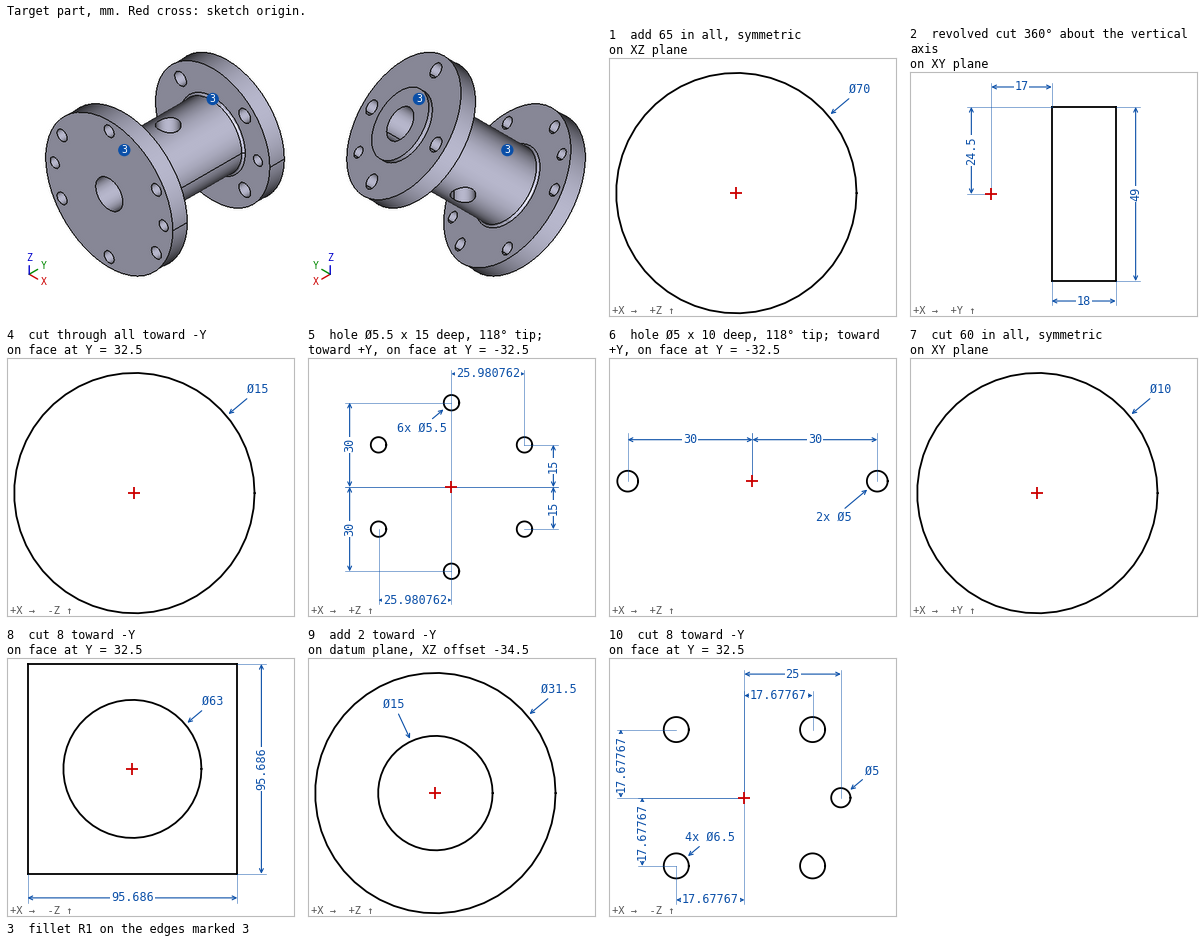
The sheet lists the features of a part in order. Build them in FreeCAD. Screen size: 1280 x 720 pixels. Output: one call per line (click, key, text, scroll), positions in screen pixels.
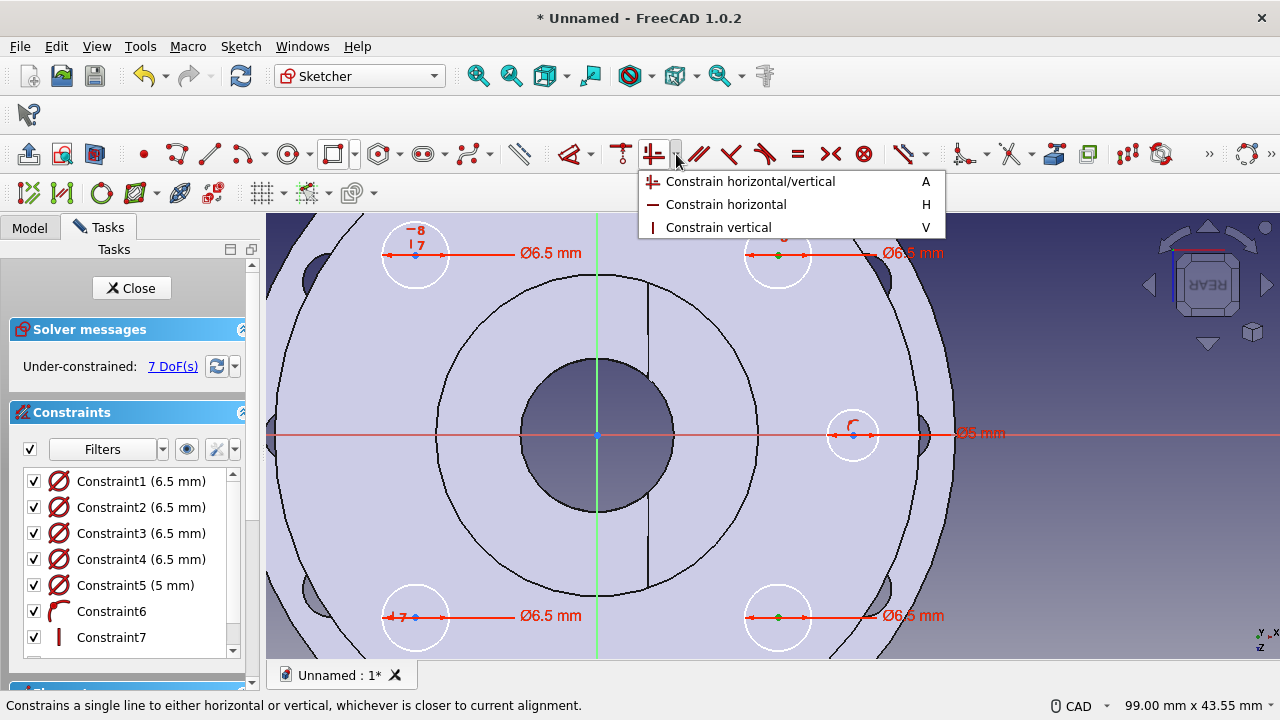
click(792, 228)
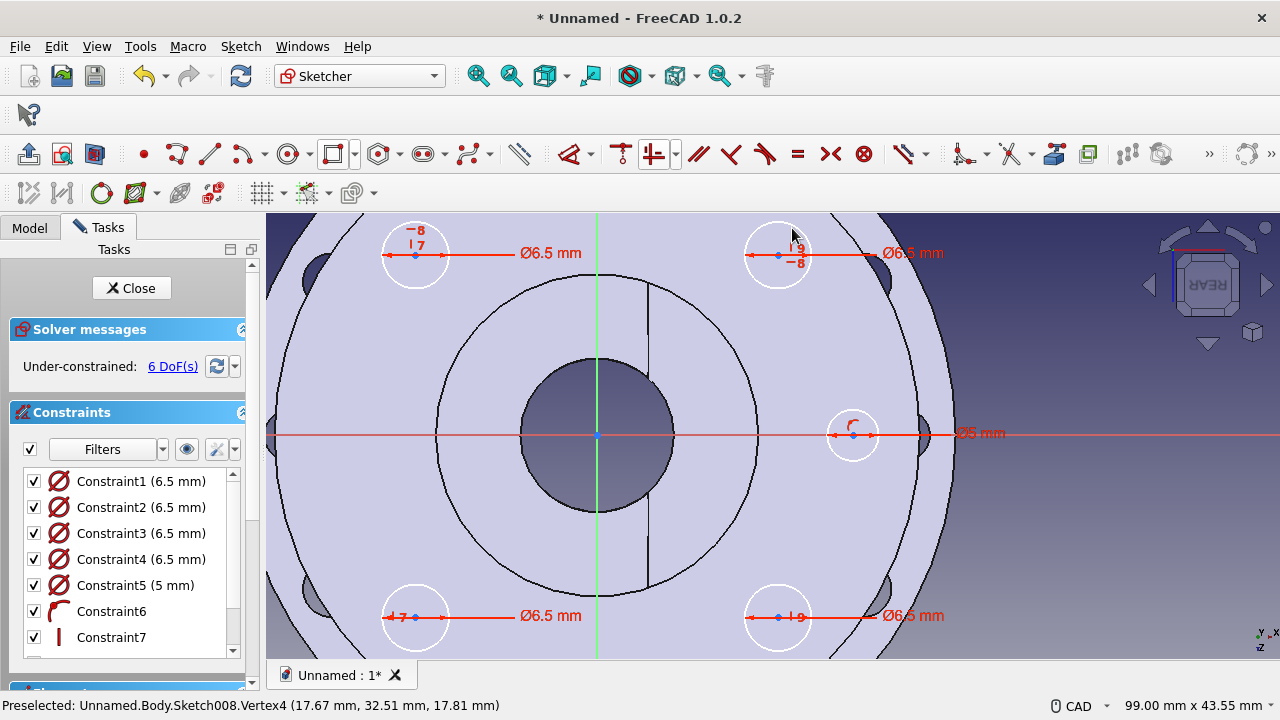
click(416, 618)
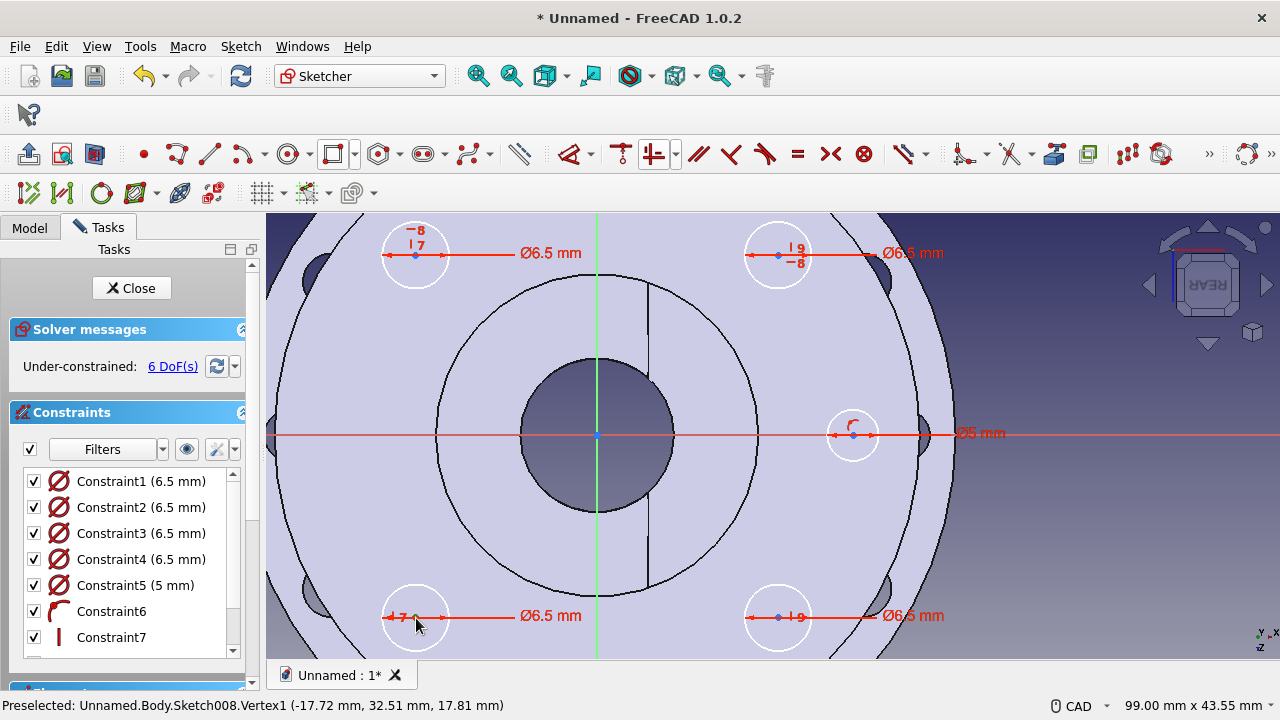
click(778, 618)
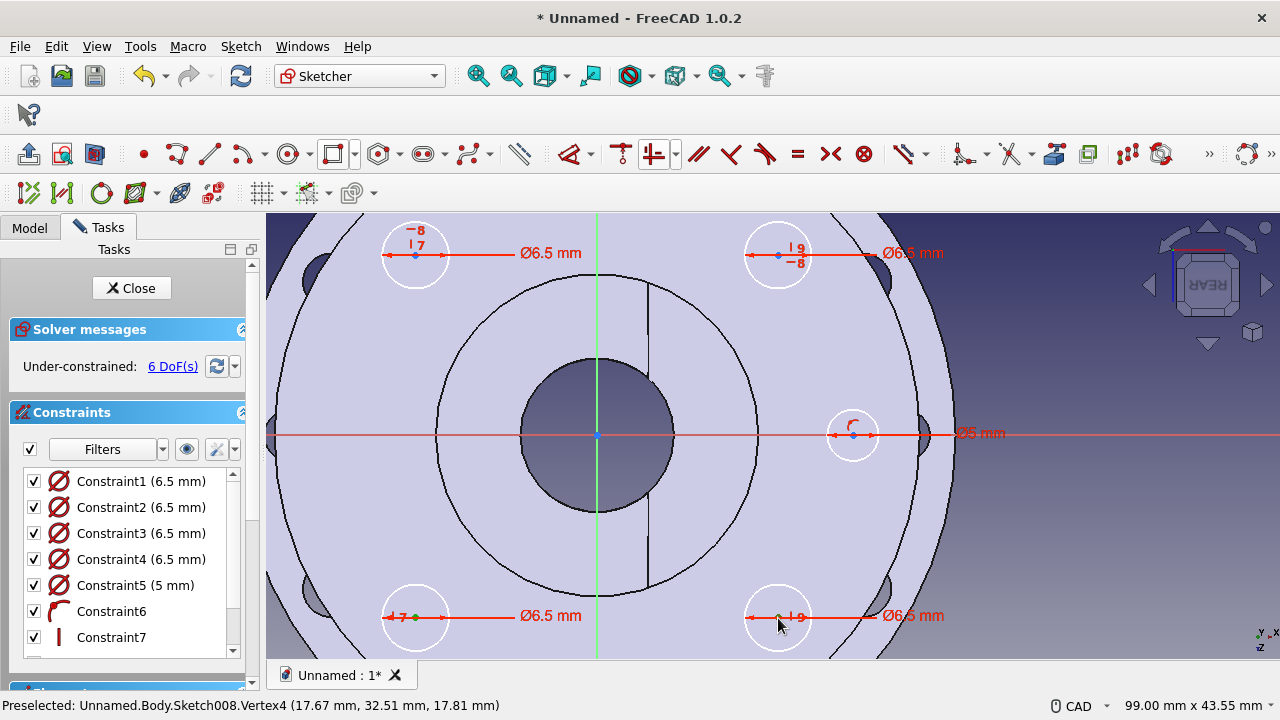
click(676, 154)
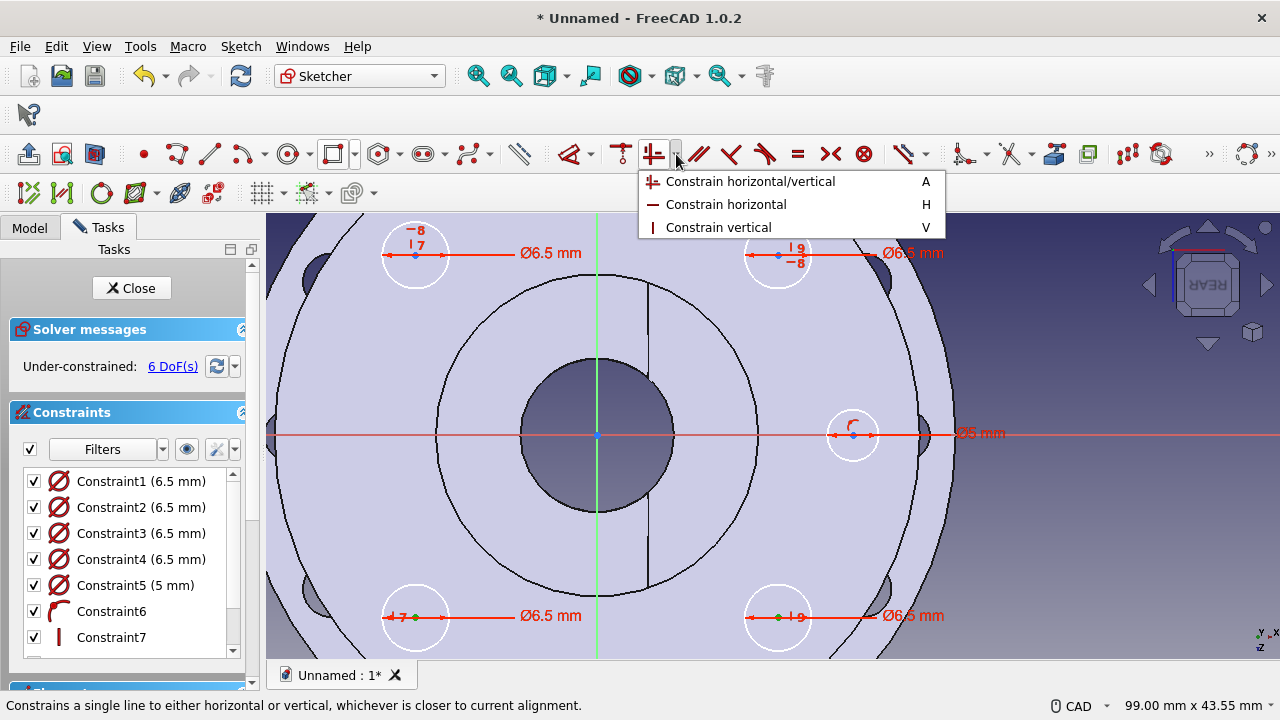
click(792, 204)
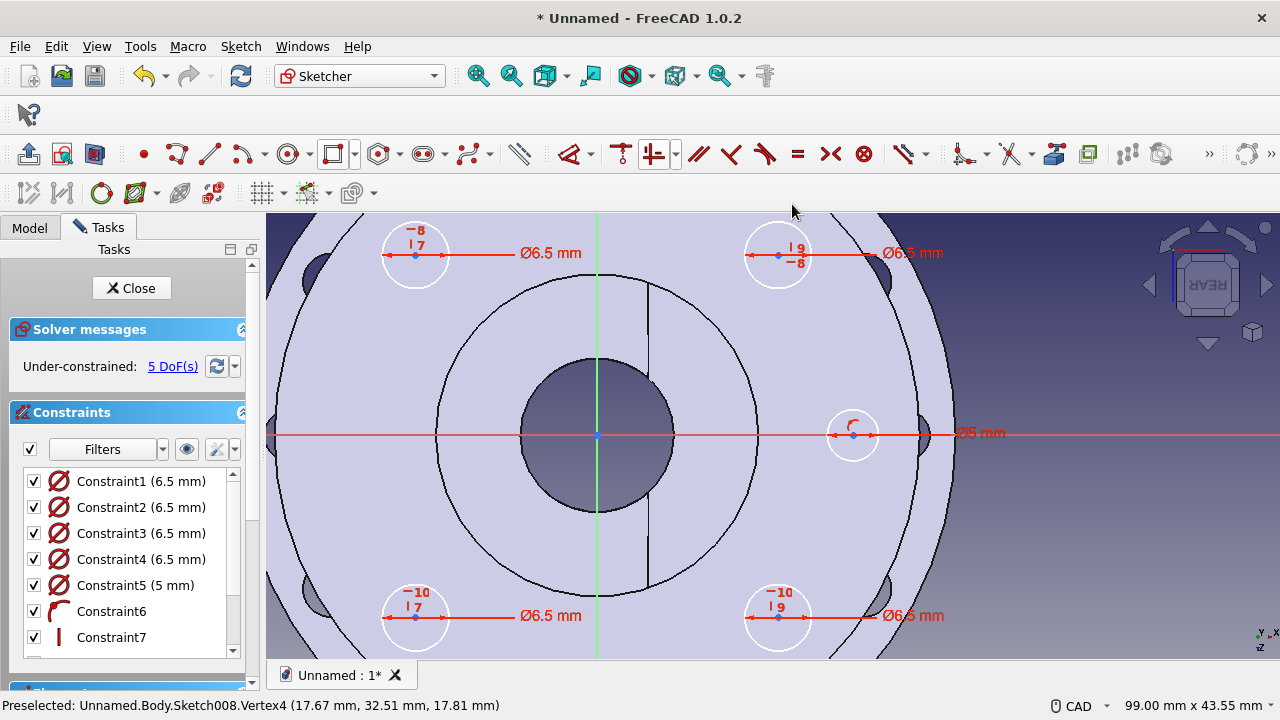
click(568, 154)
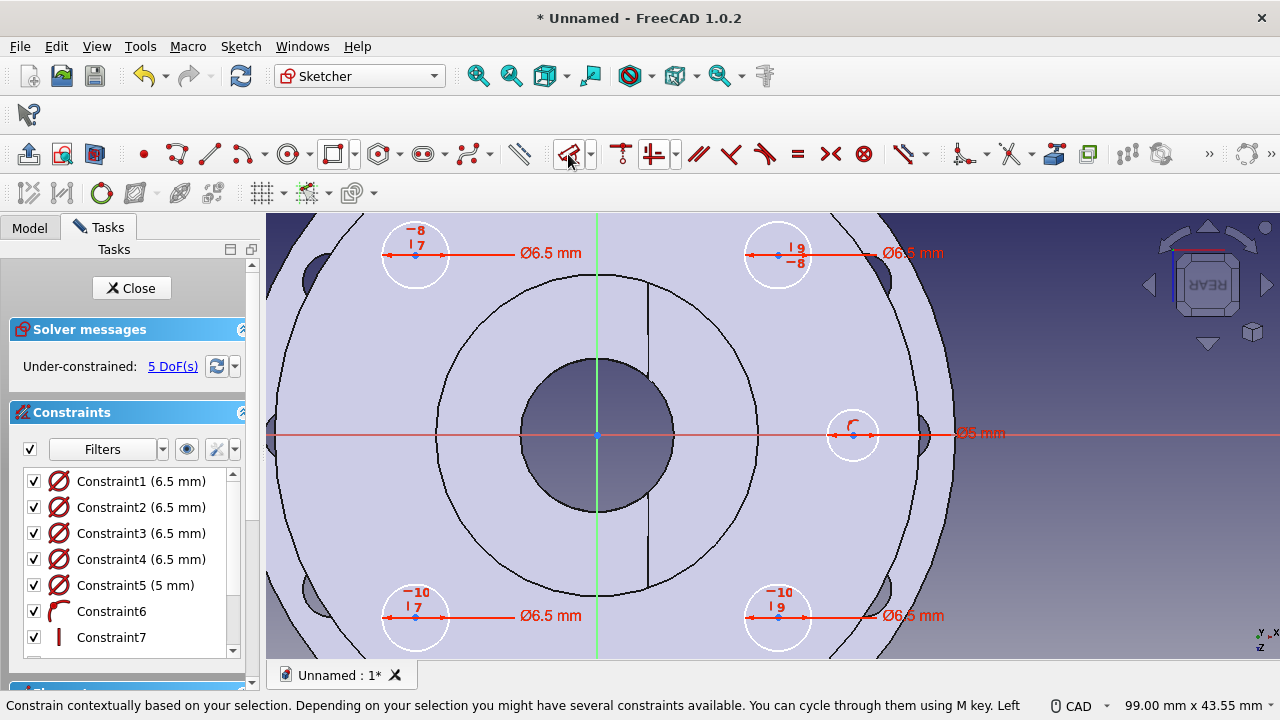
click(853, 435)
click(725, 469)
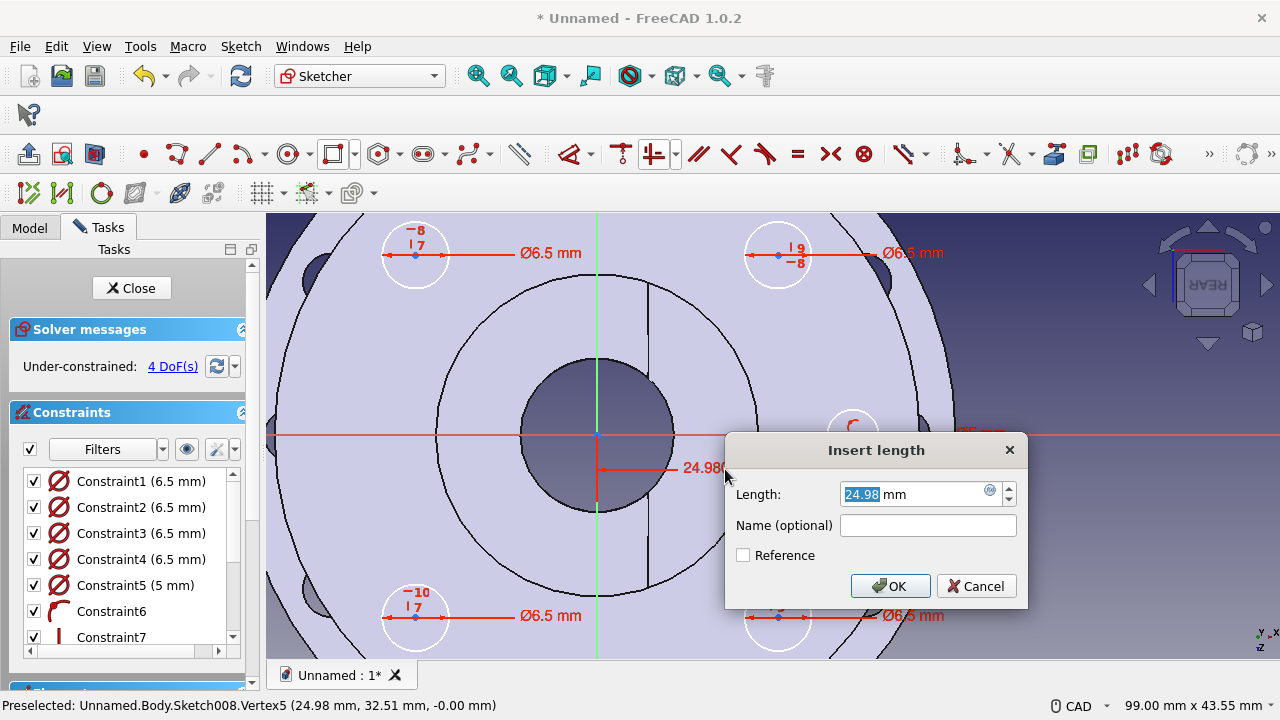
text(25)
key(Return)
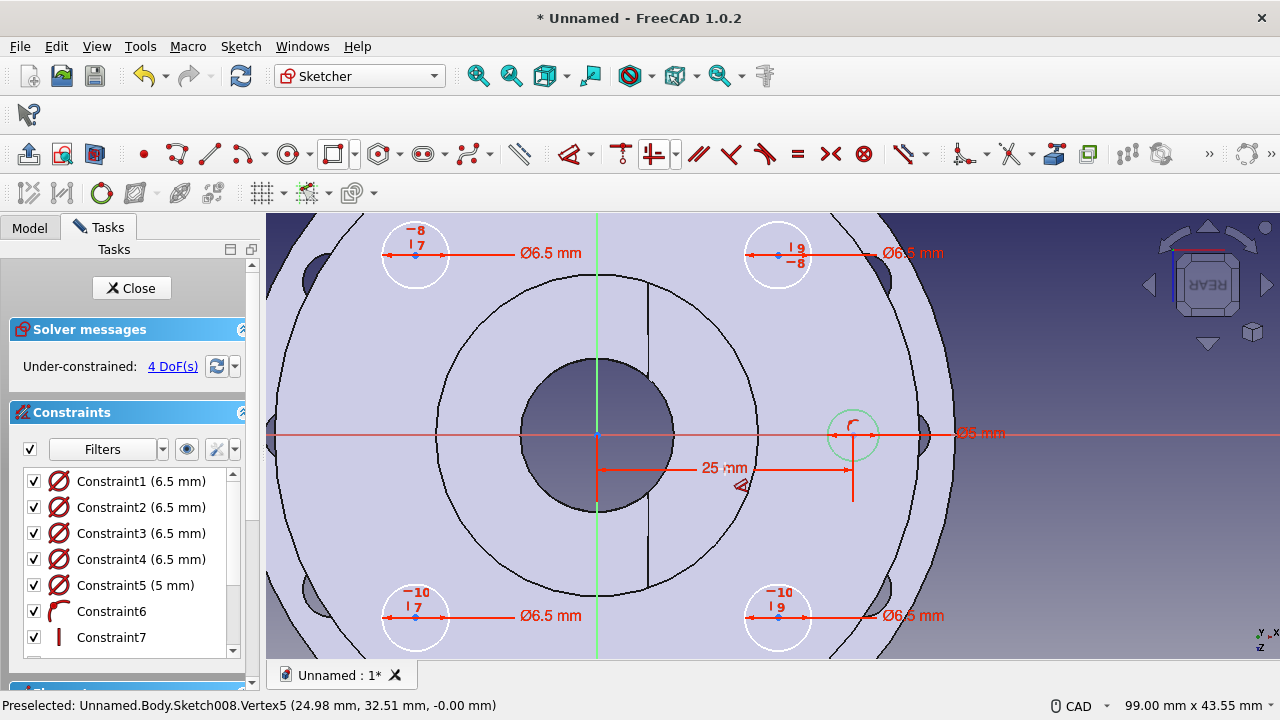
click(416, 618)
click(506, 401)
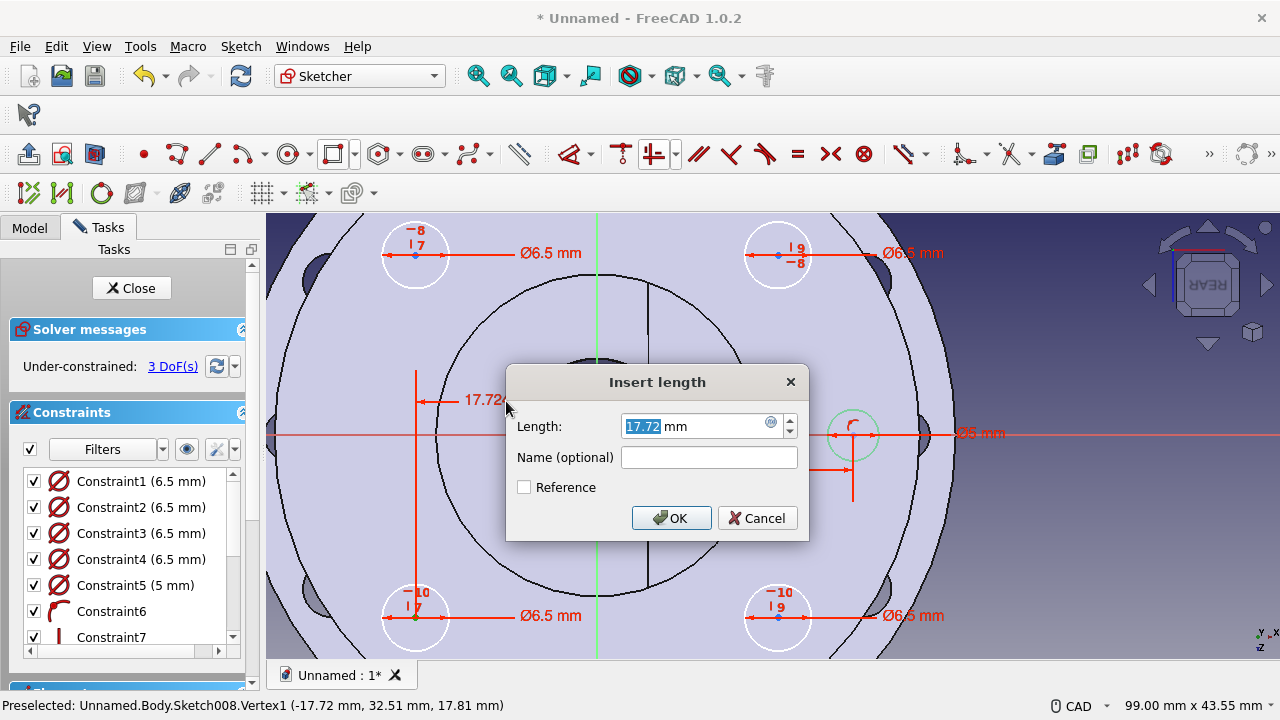
text(17.67767)
key(Return)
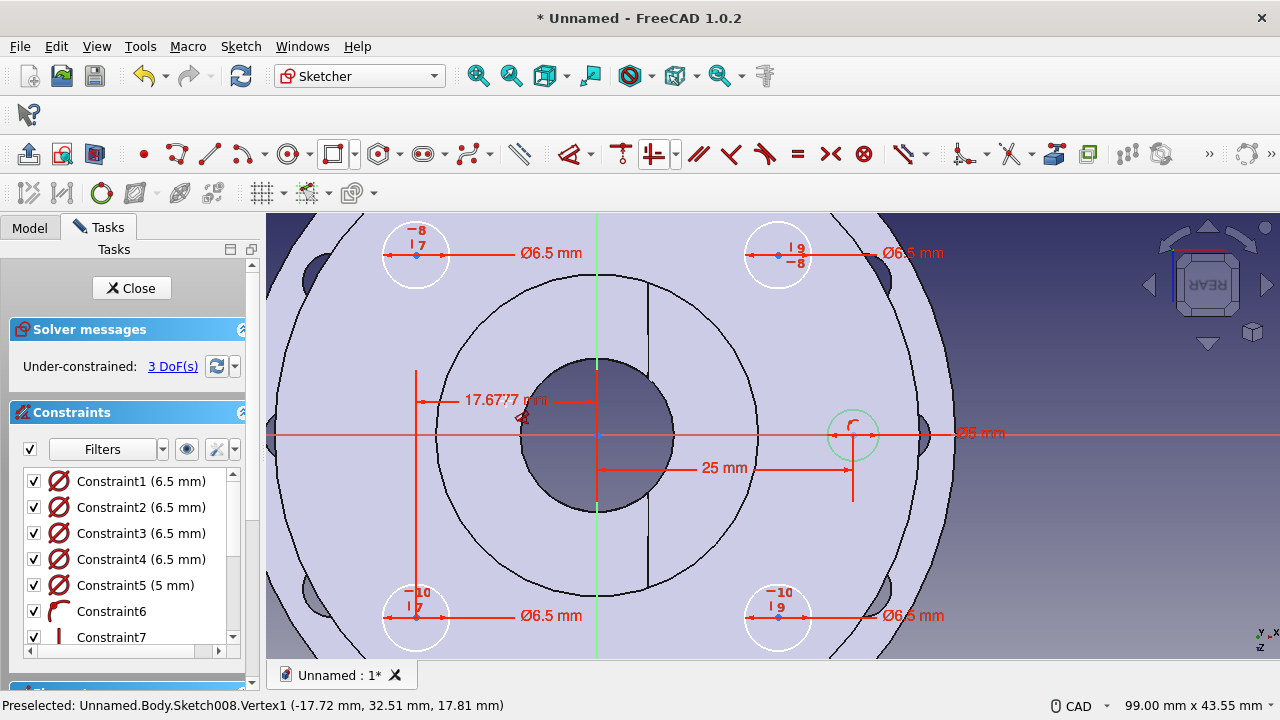
click(416, 618)
click(382, 527)